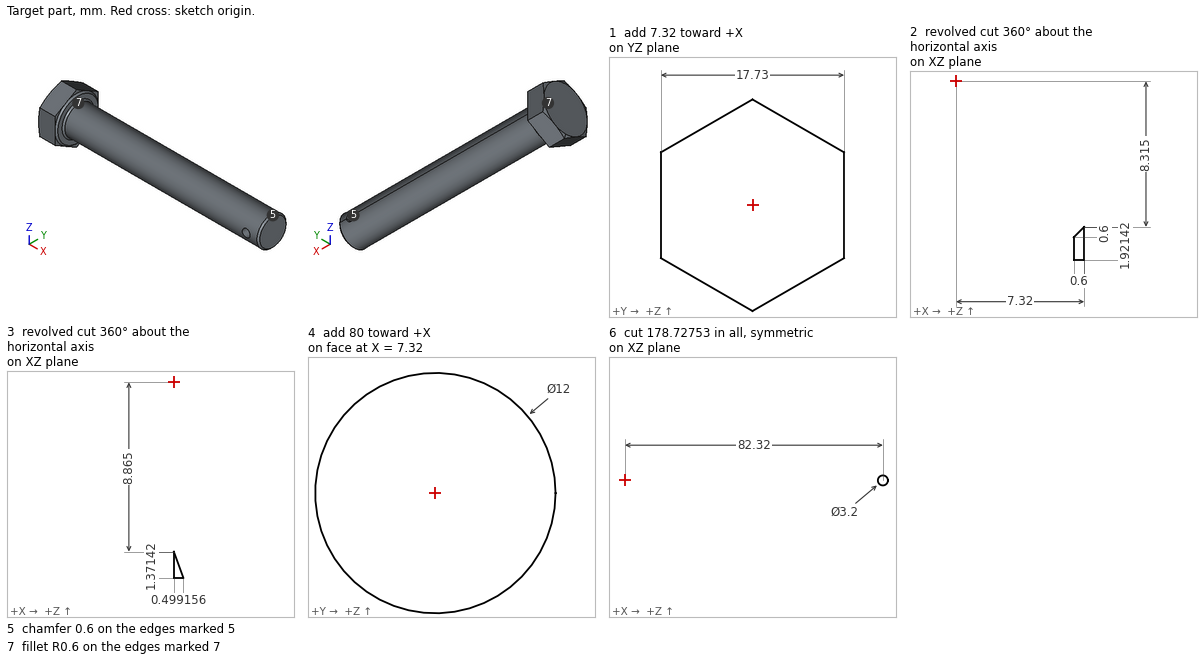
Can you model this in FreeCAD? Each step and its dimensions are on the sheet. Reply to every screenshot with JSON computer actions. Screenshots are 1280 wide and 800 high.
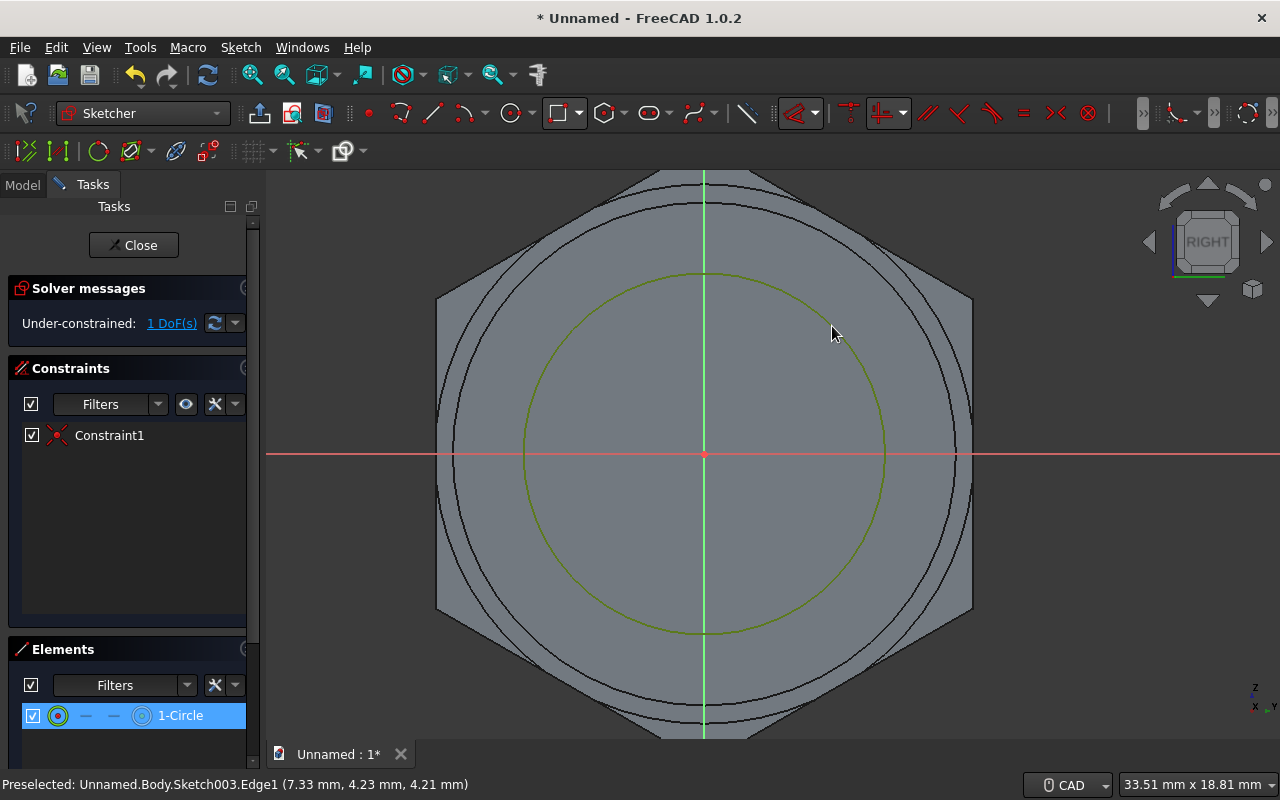
{"action": "left_click", "coordinate": [818, 114]}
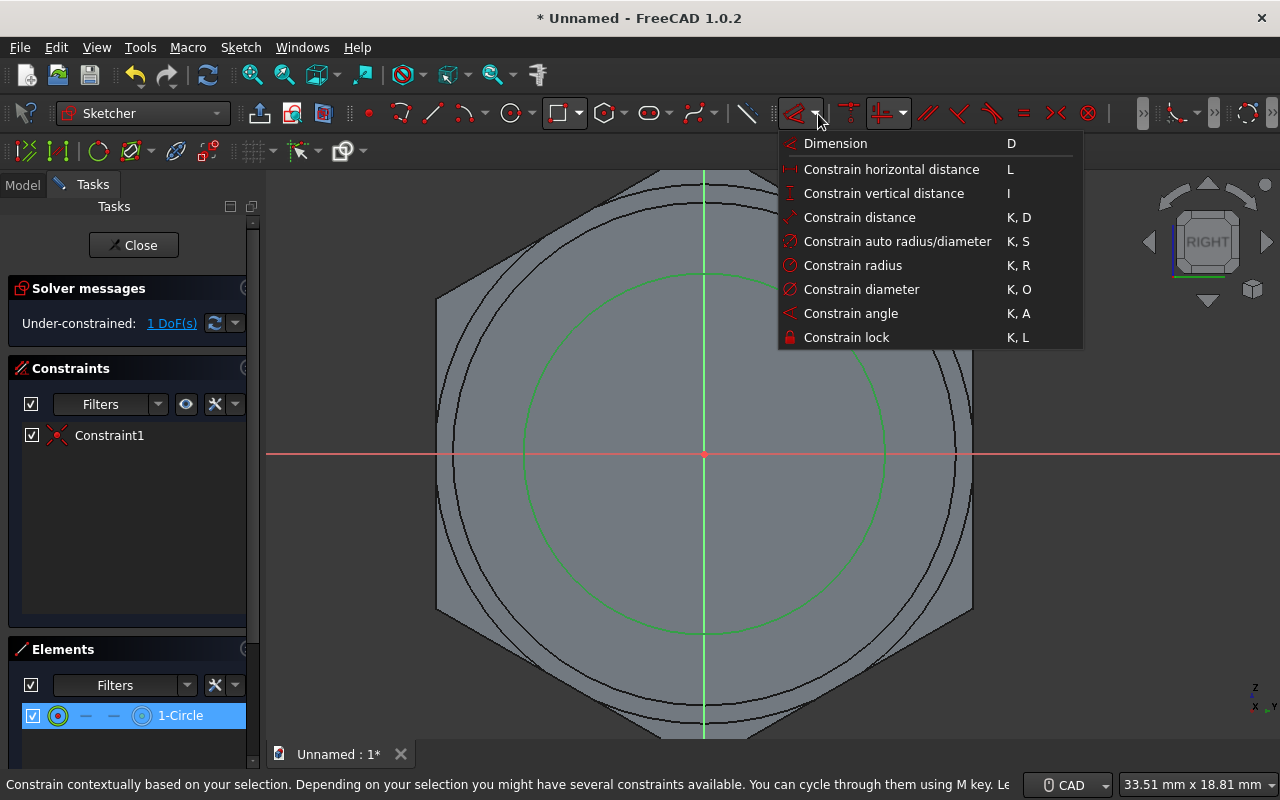
{"action": "left_click", "coordinate": [931, 289]}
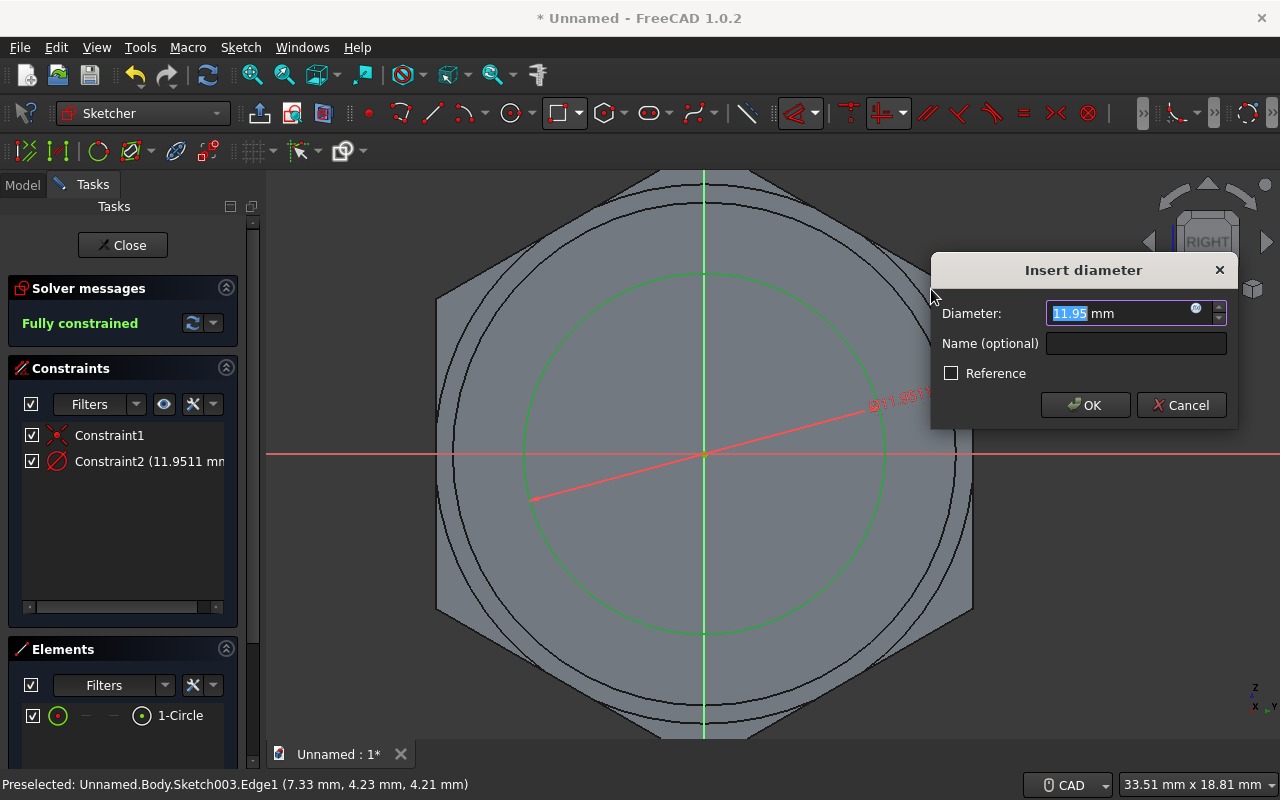
{"action": "type", "text": "12"}
{"action": "key", "text": "Return"}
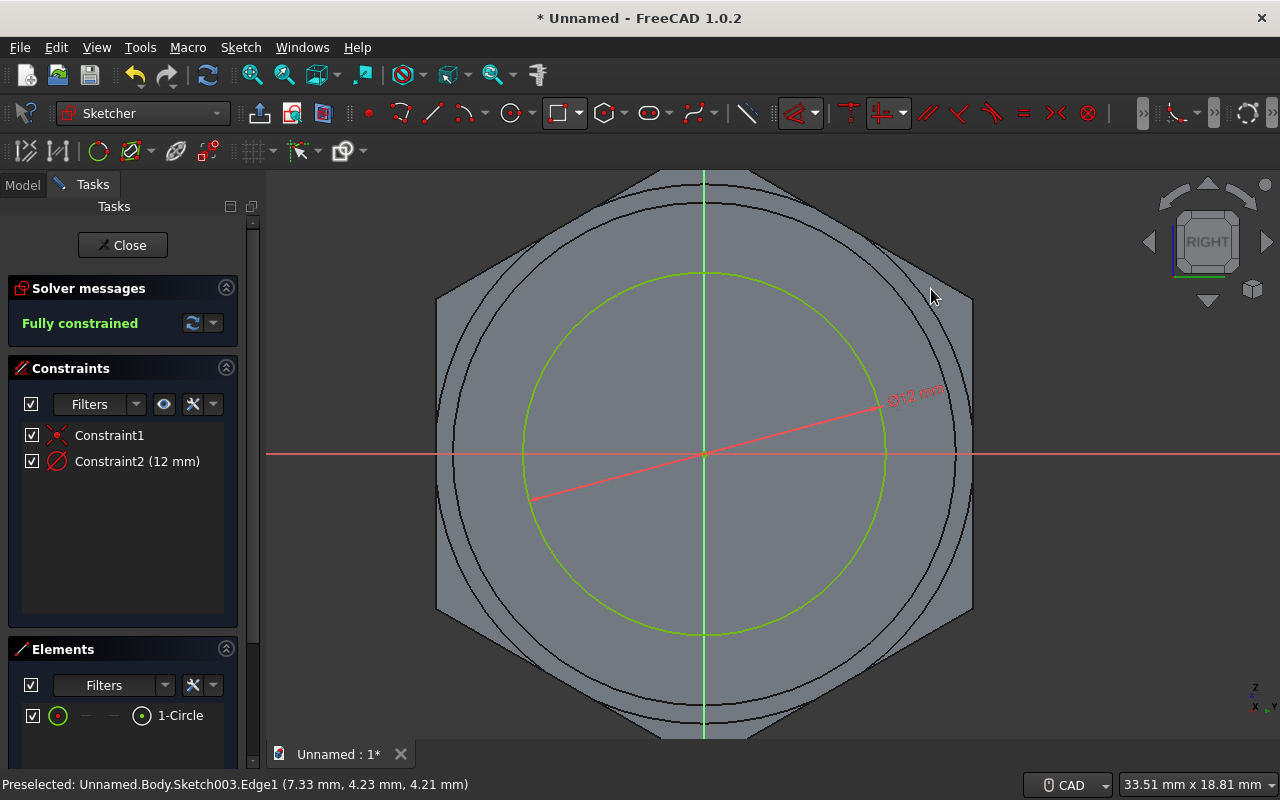
{"action": "left_click", "coordinate": [123, 245]}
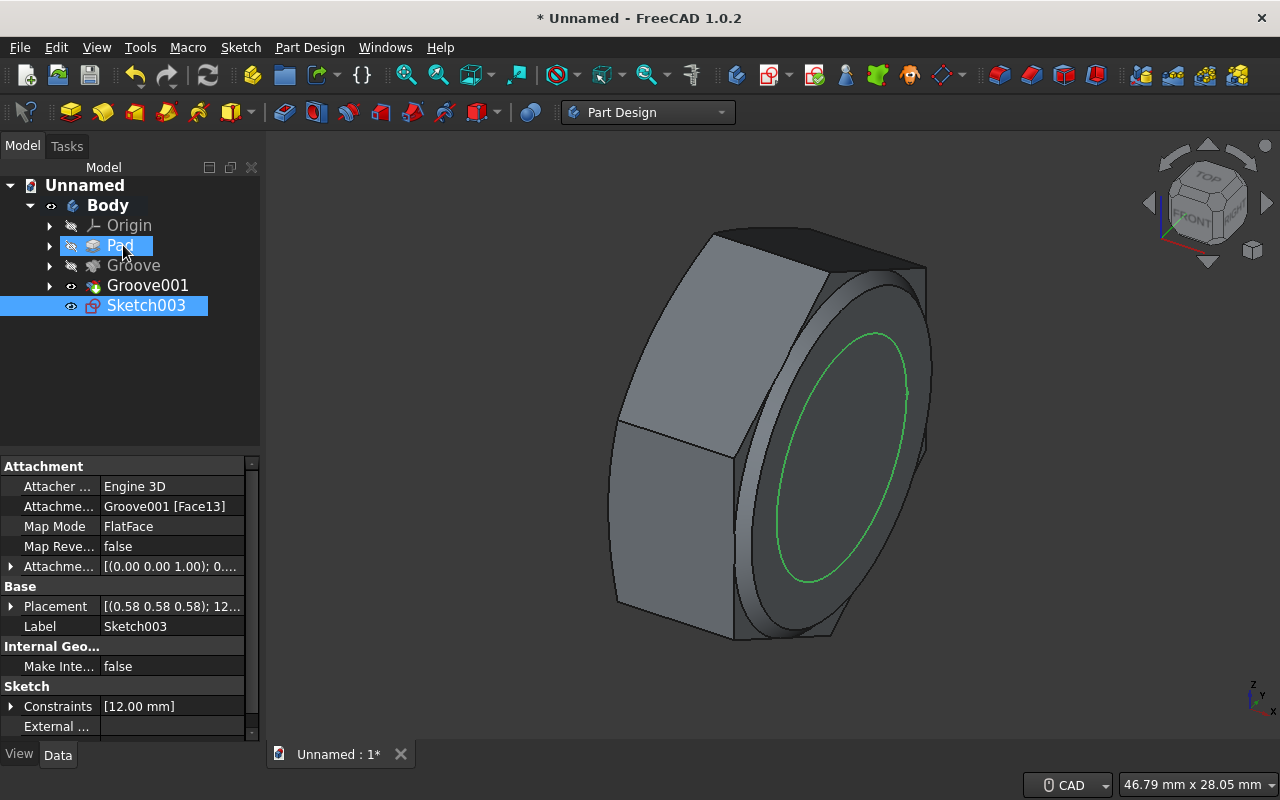
{"action": "left_click", "coordinate": [72, 112]}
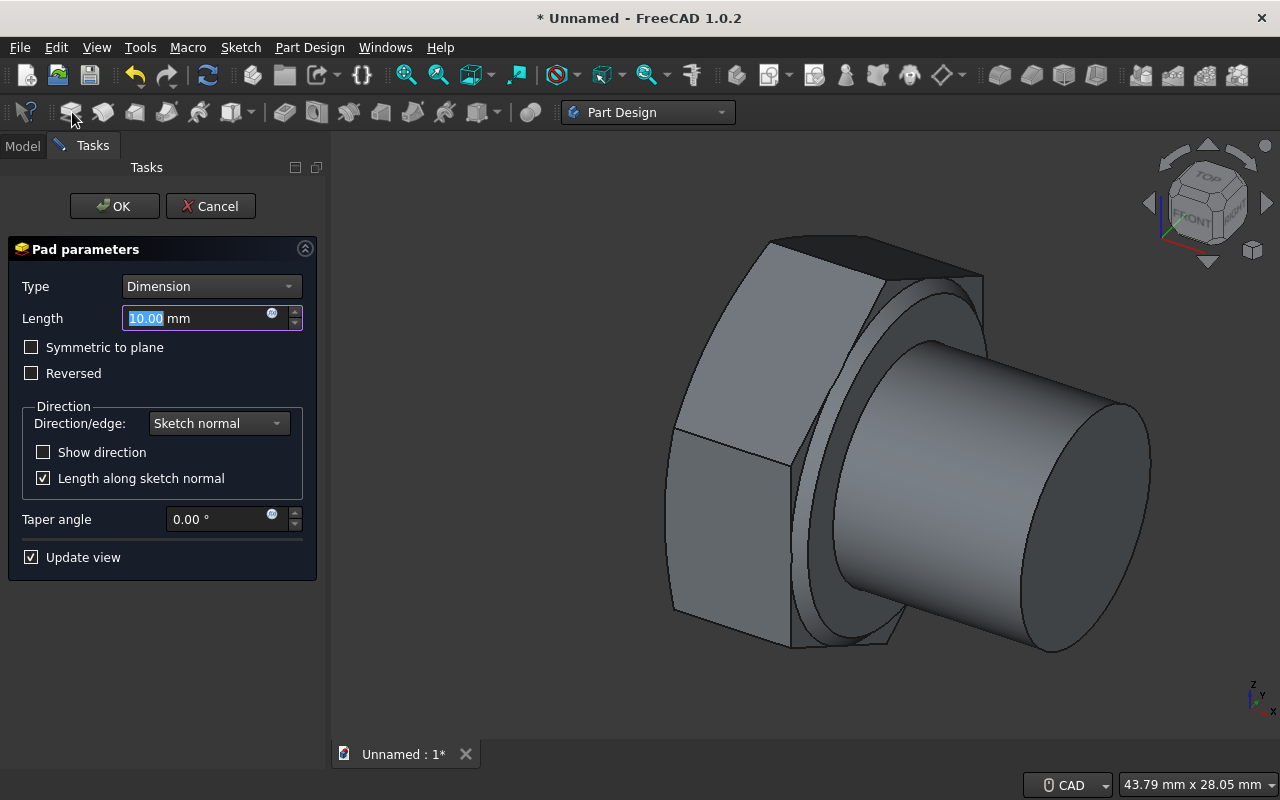
{"action": "type", "text": "80"}
{"action": "key", "text": "Tab"}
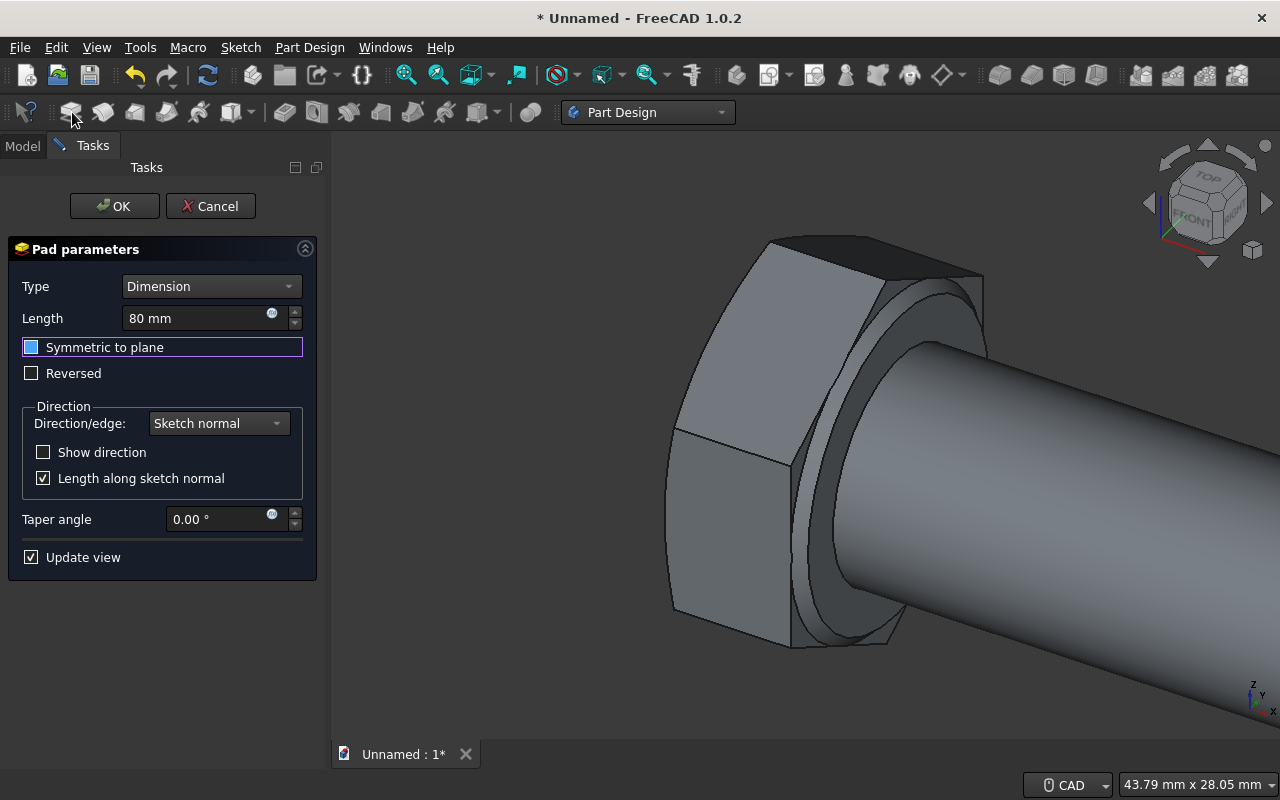
{"action": "left_click", "coordinate": [115, 206]}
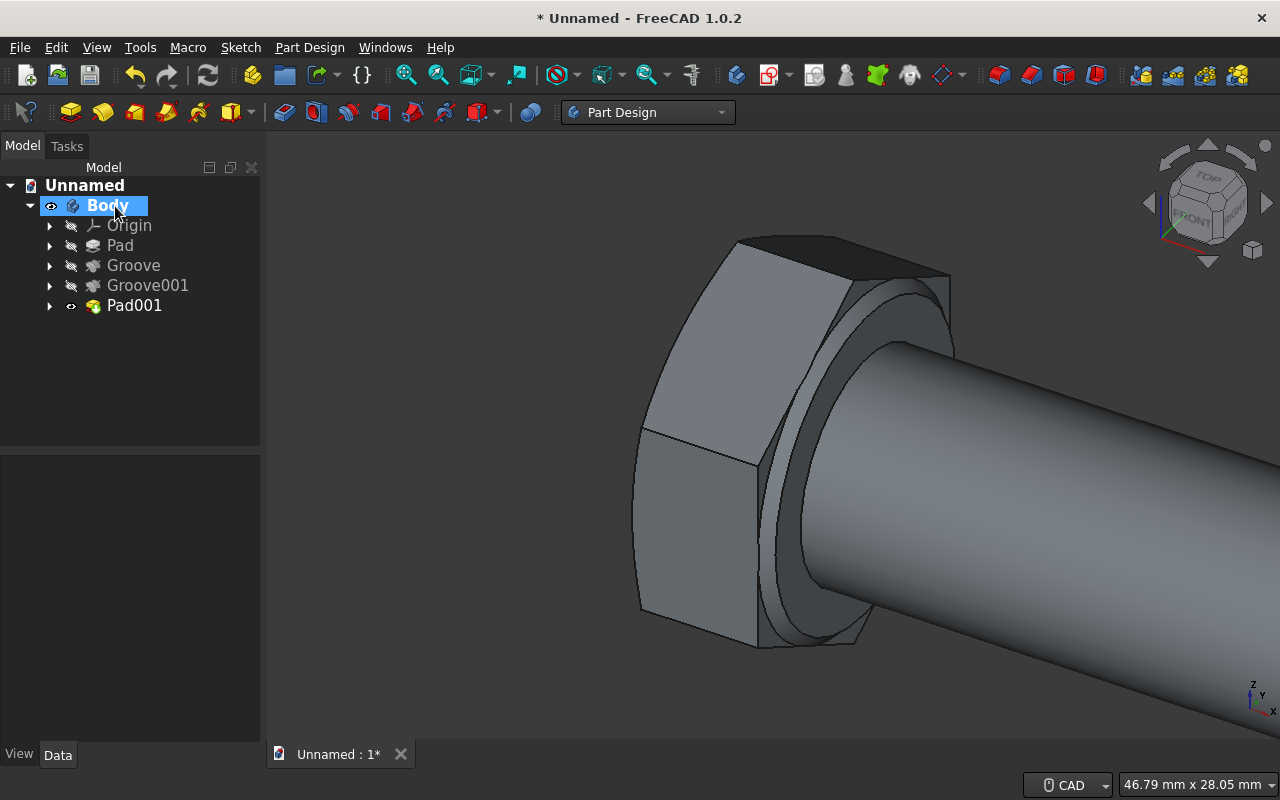
{"action": "left_click", "coordinate": [408, 76]}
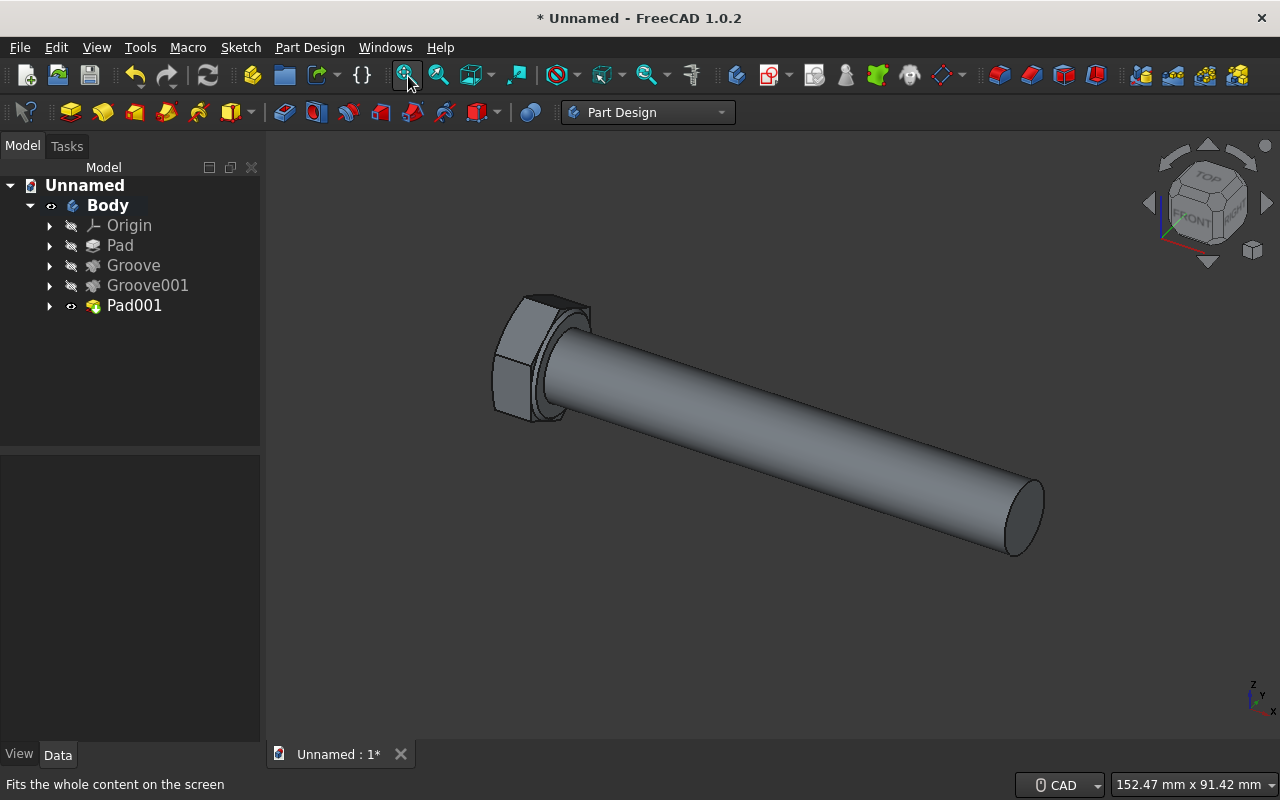
{"action": "left_click", "coordinate": [1005, 537]}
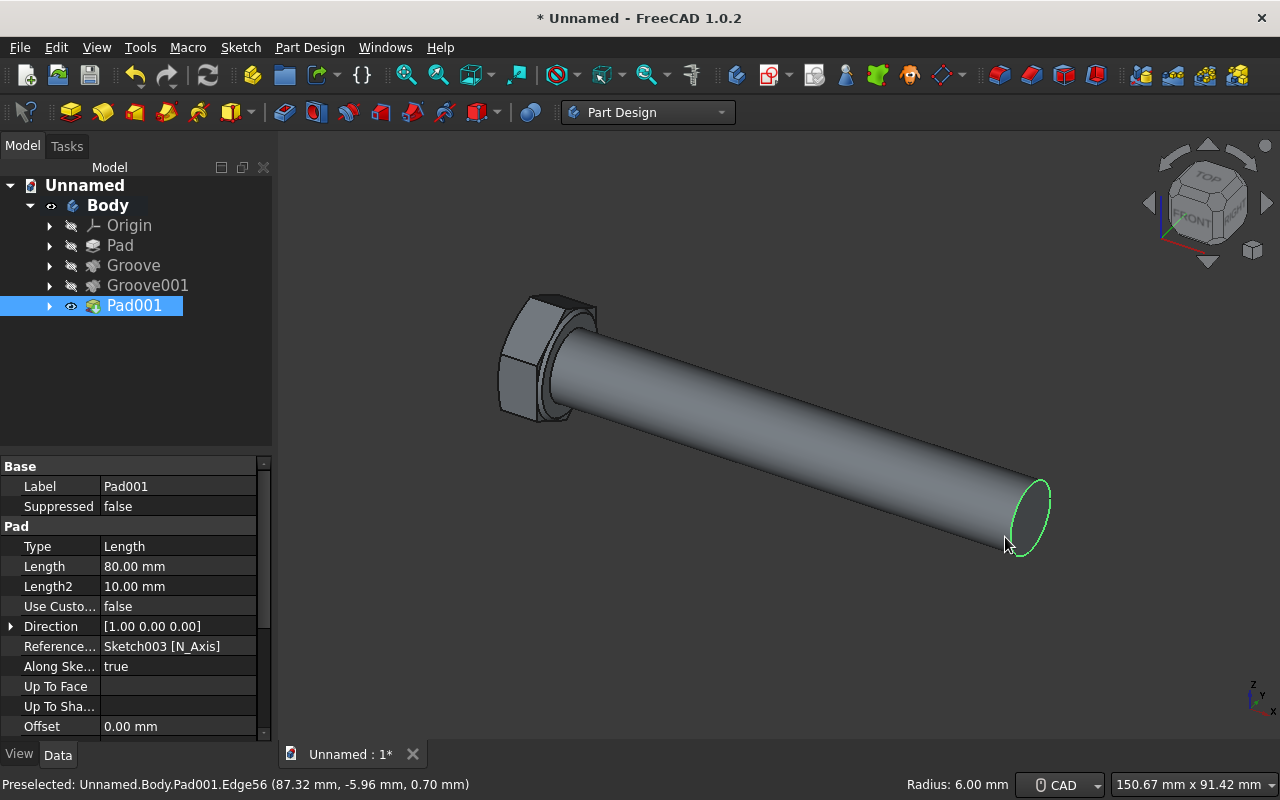
{"action": "left_click", "coordinate": [1032, 76]}